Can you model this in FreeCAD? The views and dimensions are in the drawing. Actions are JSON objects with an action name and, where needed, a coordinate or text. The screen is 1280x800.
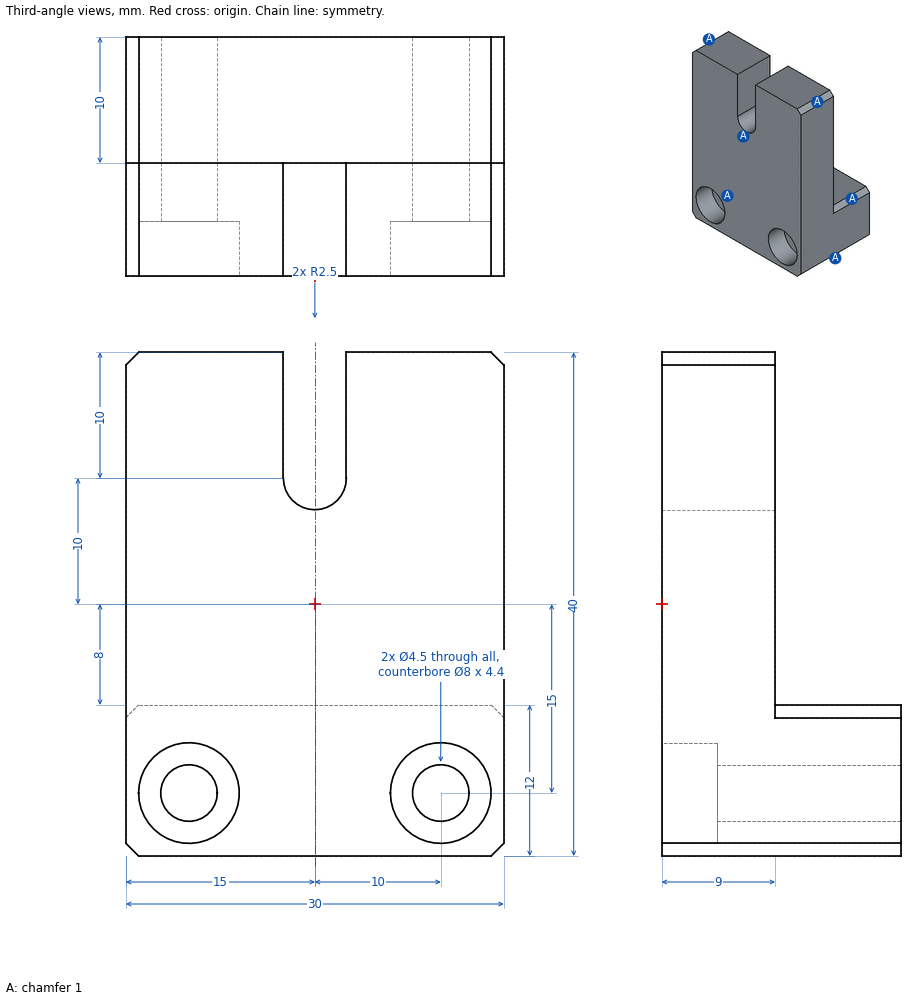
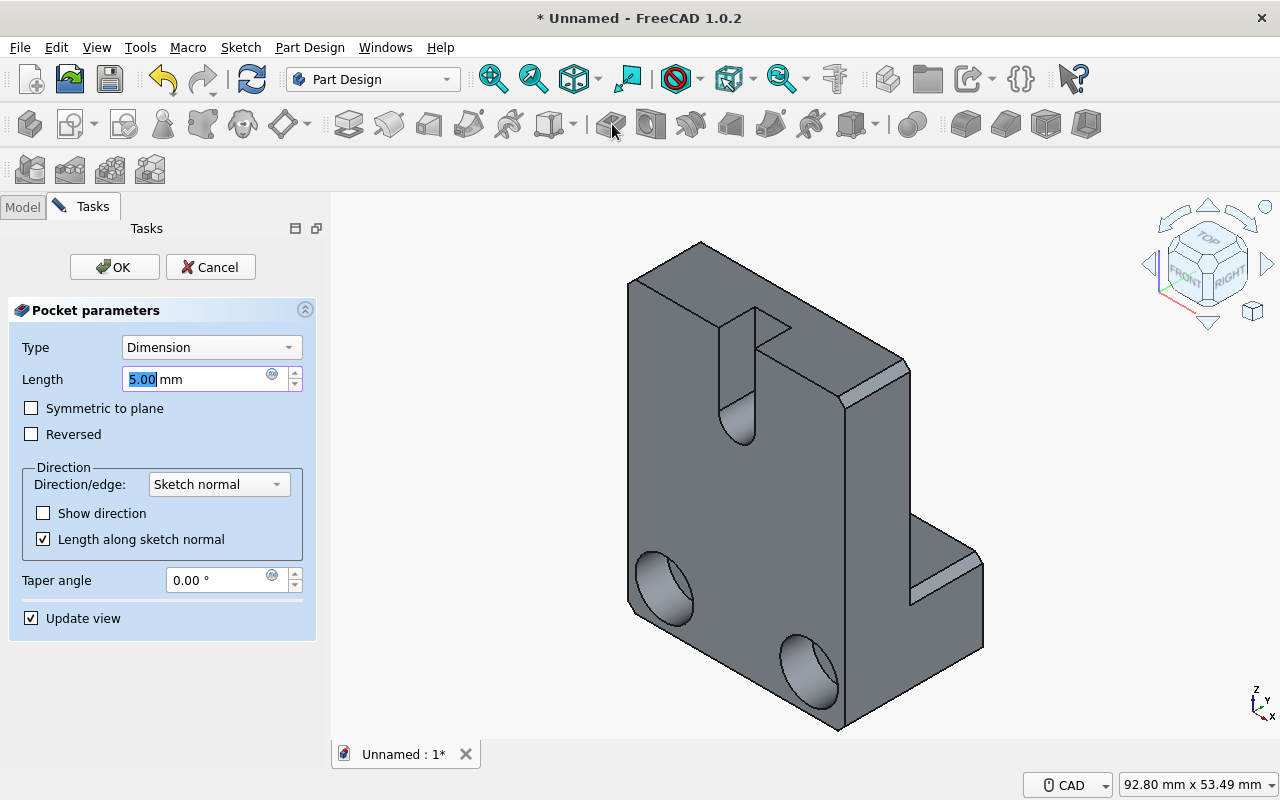
{"action": "left_click", "coordinate": [212, 348]}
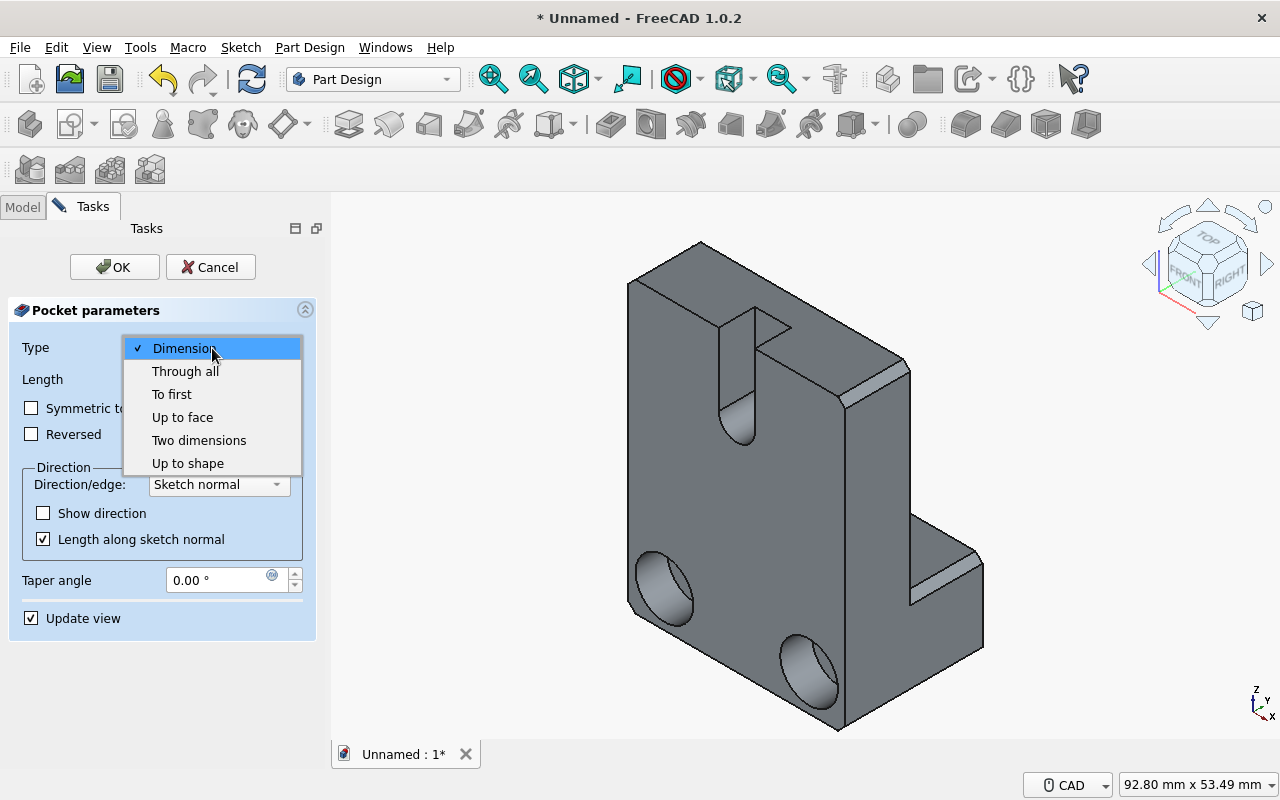
{"action": "left_click", "coordinate": [212, 372]}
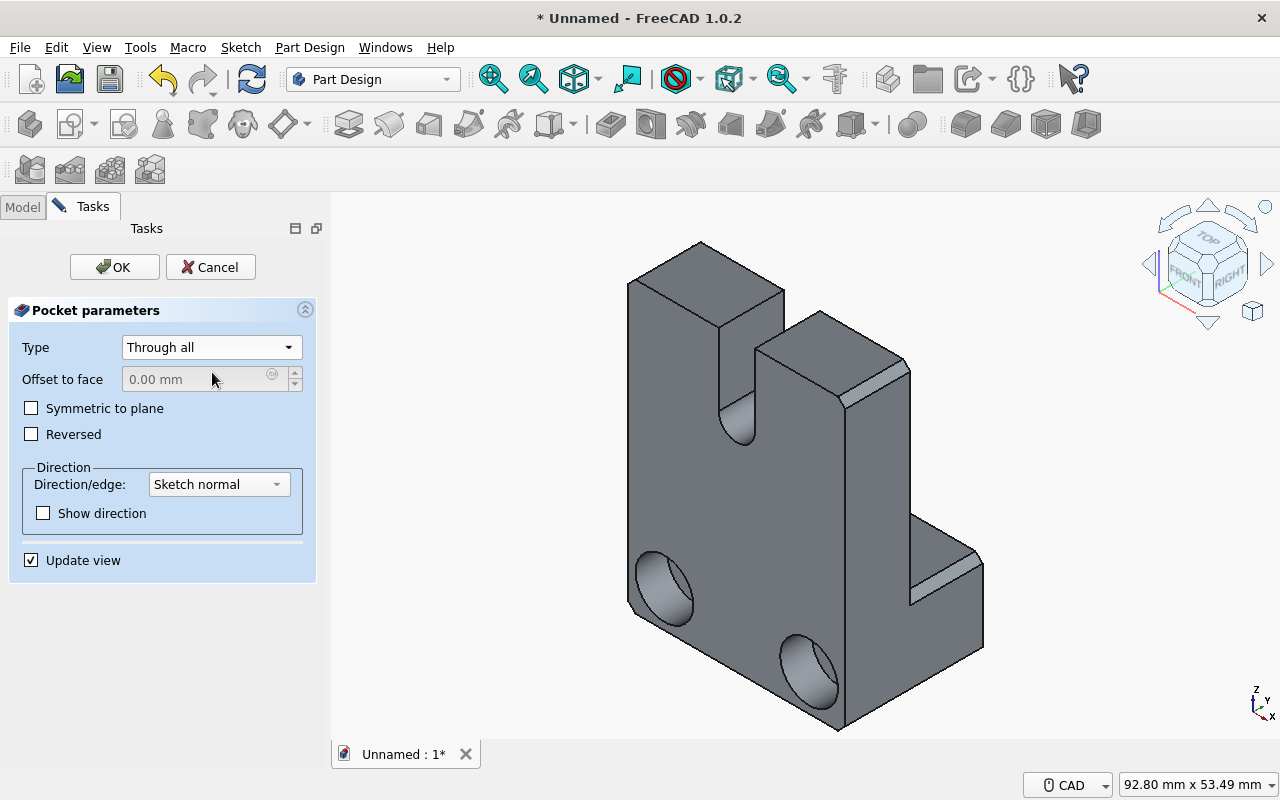
{"action": "left_click", "coordinate": [115, 267]}